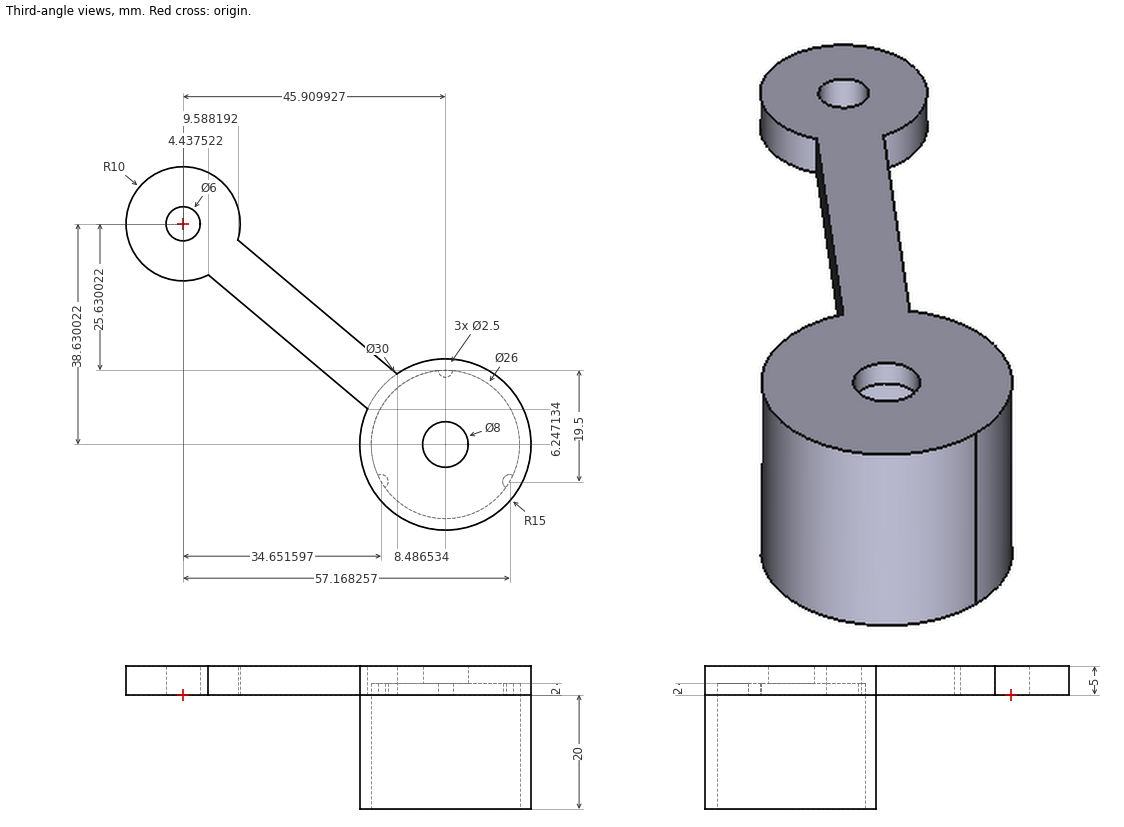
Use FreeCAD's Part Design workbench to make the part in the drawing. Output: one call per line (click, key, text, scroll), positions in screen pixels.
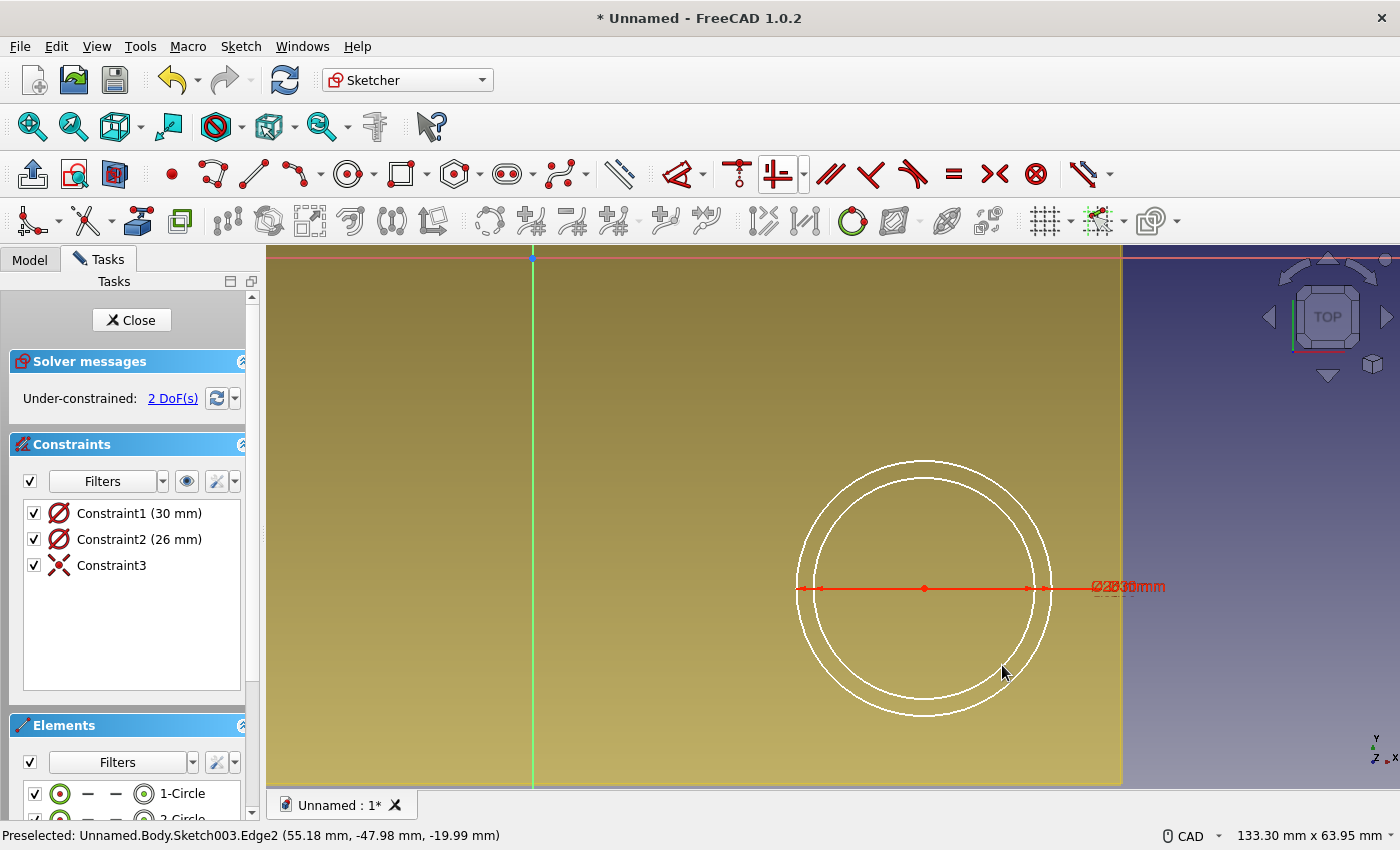
key(d)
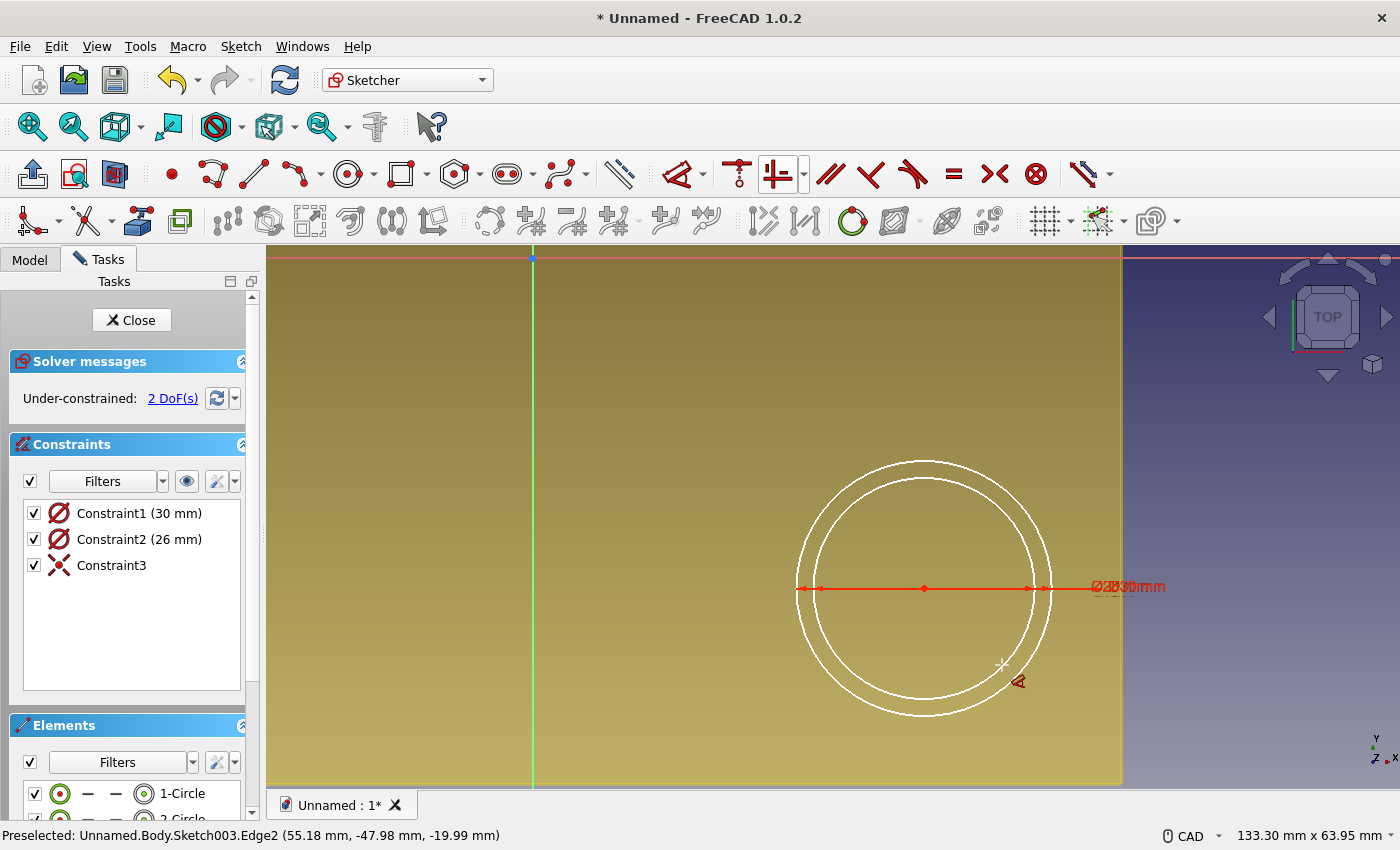
click(924, 589)
click(729, 623)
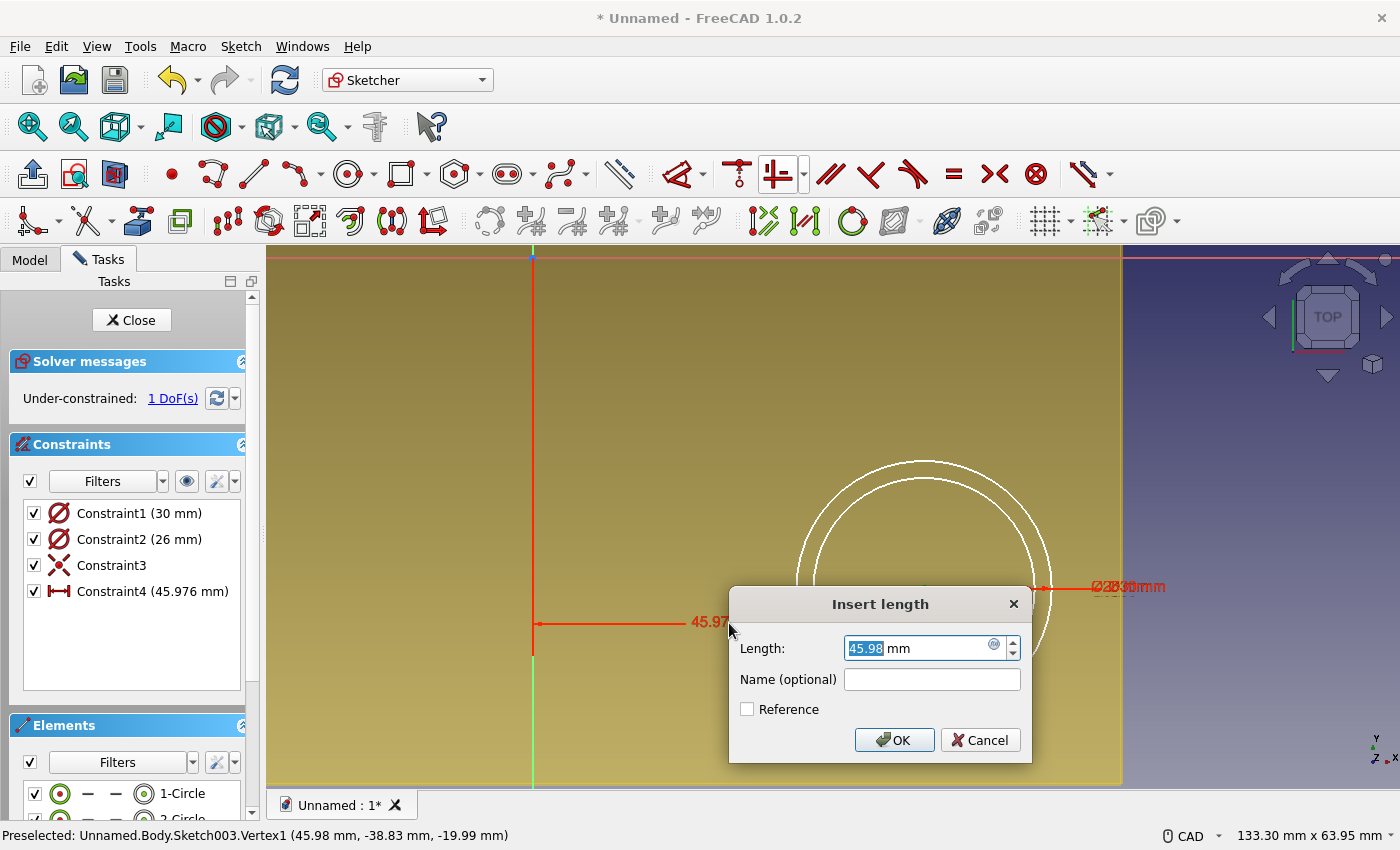
text(45.909927)
key(Return)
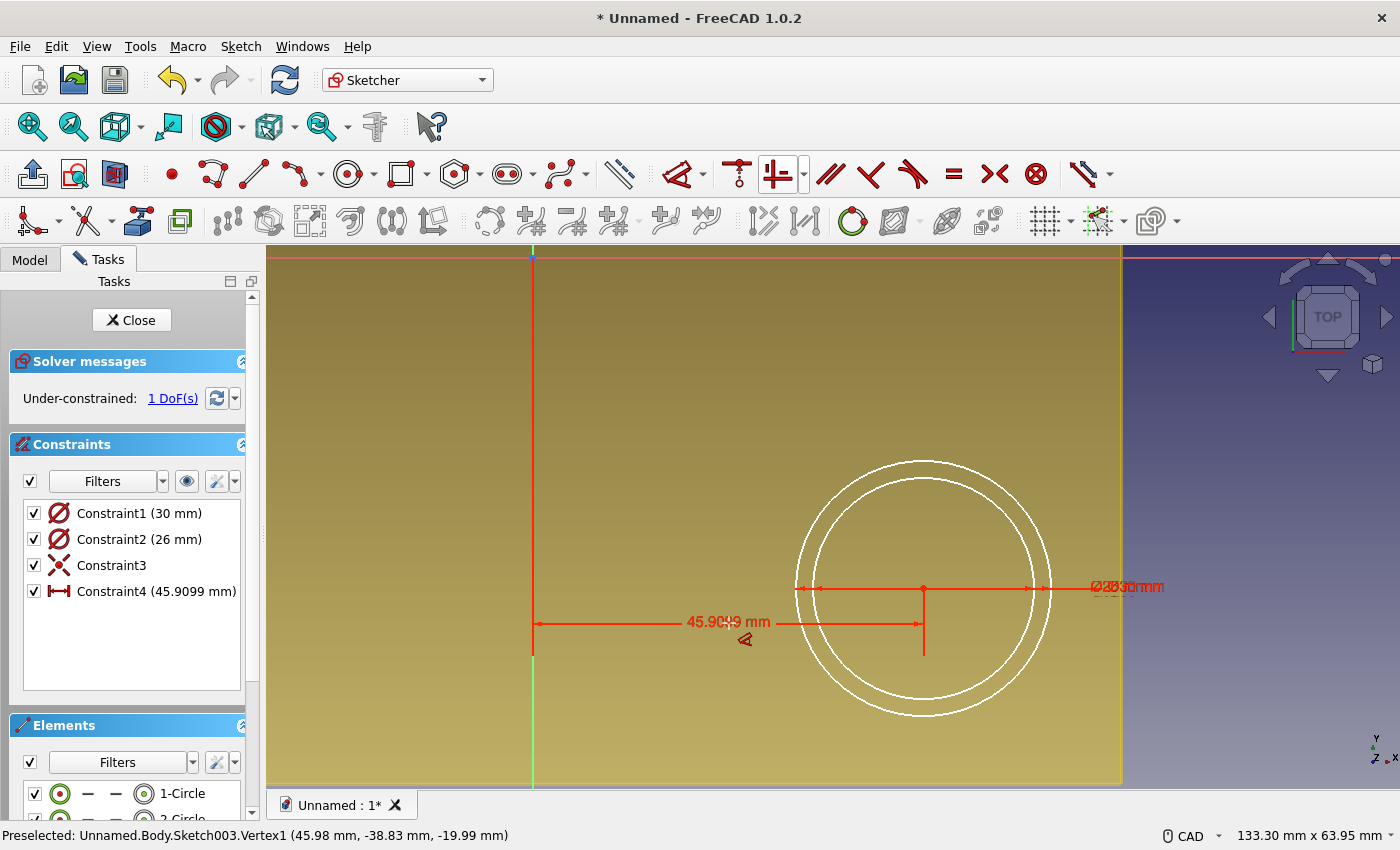
click(924, 589)
click(499, 431)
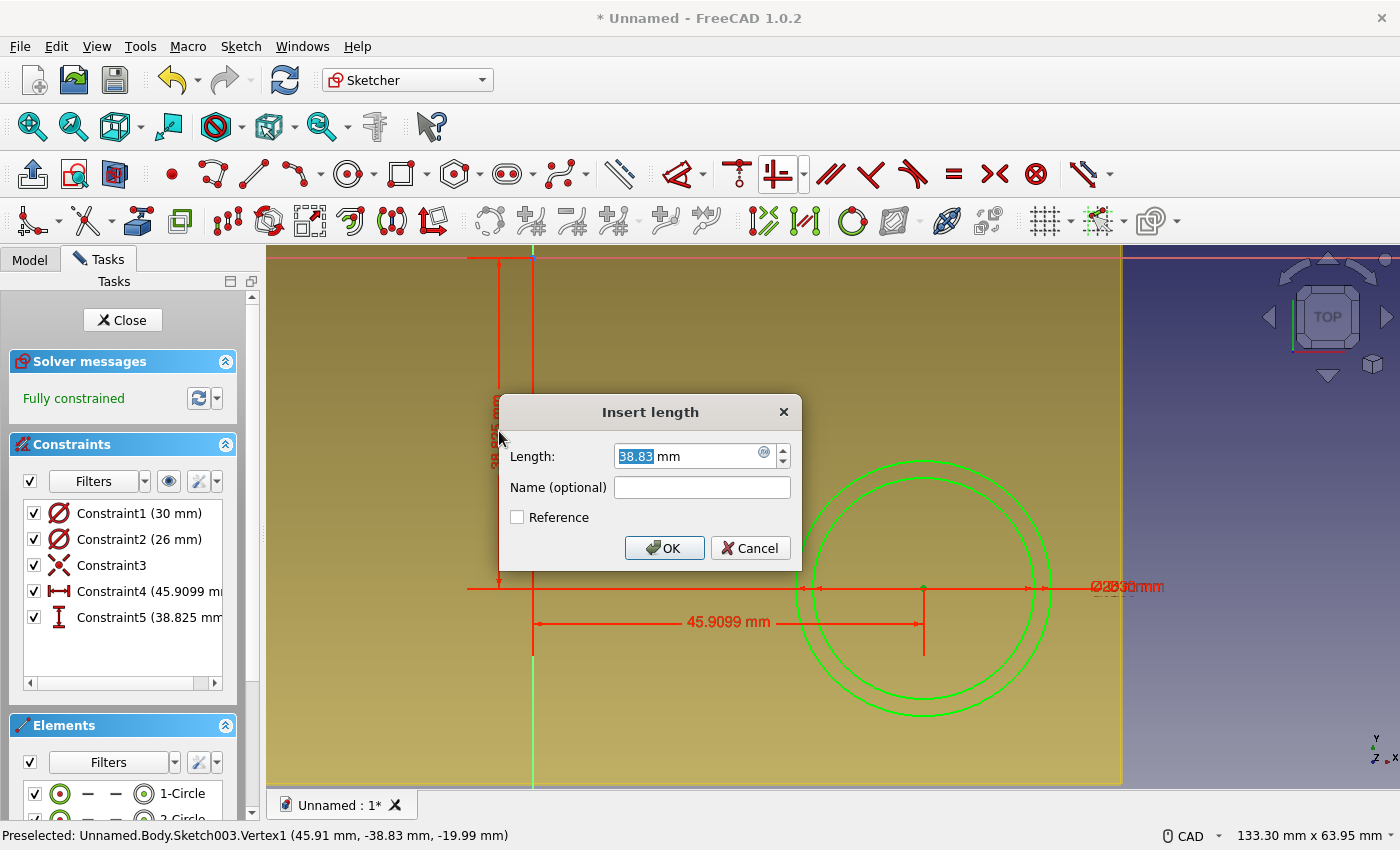
text(38.630022)
key(Return)
key(Escape)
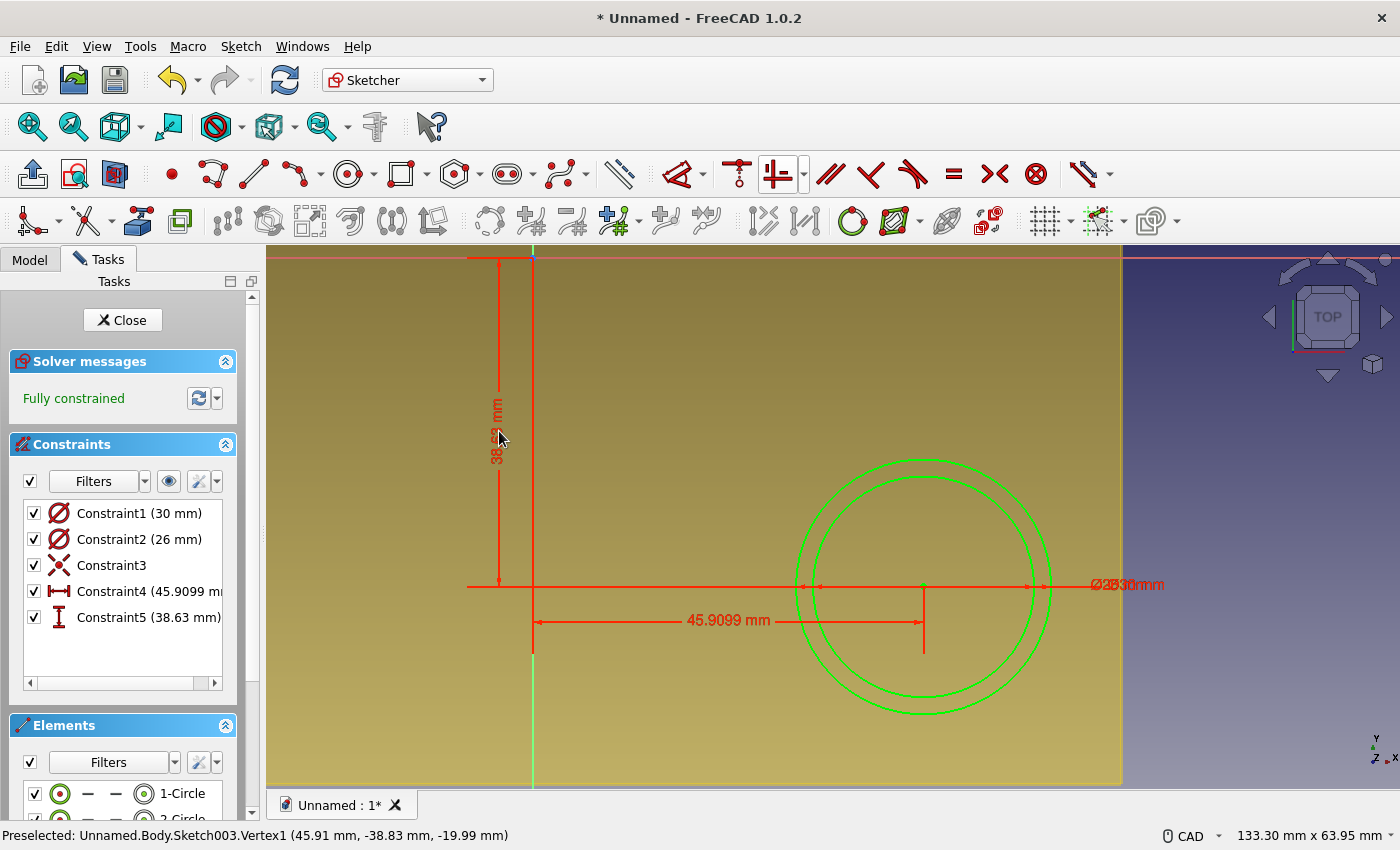
click(123, 320)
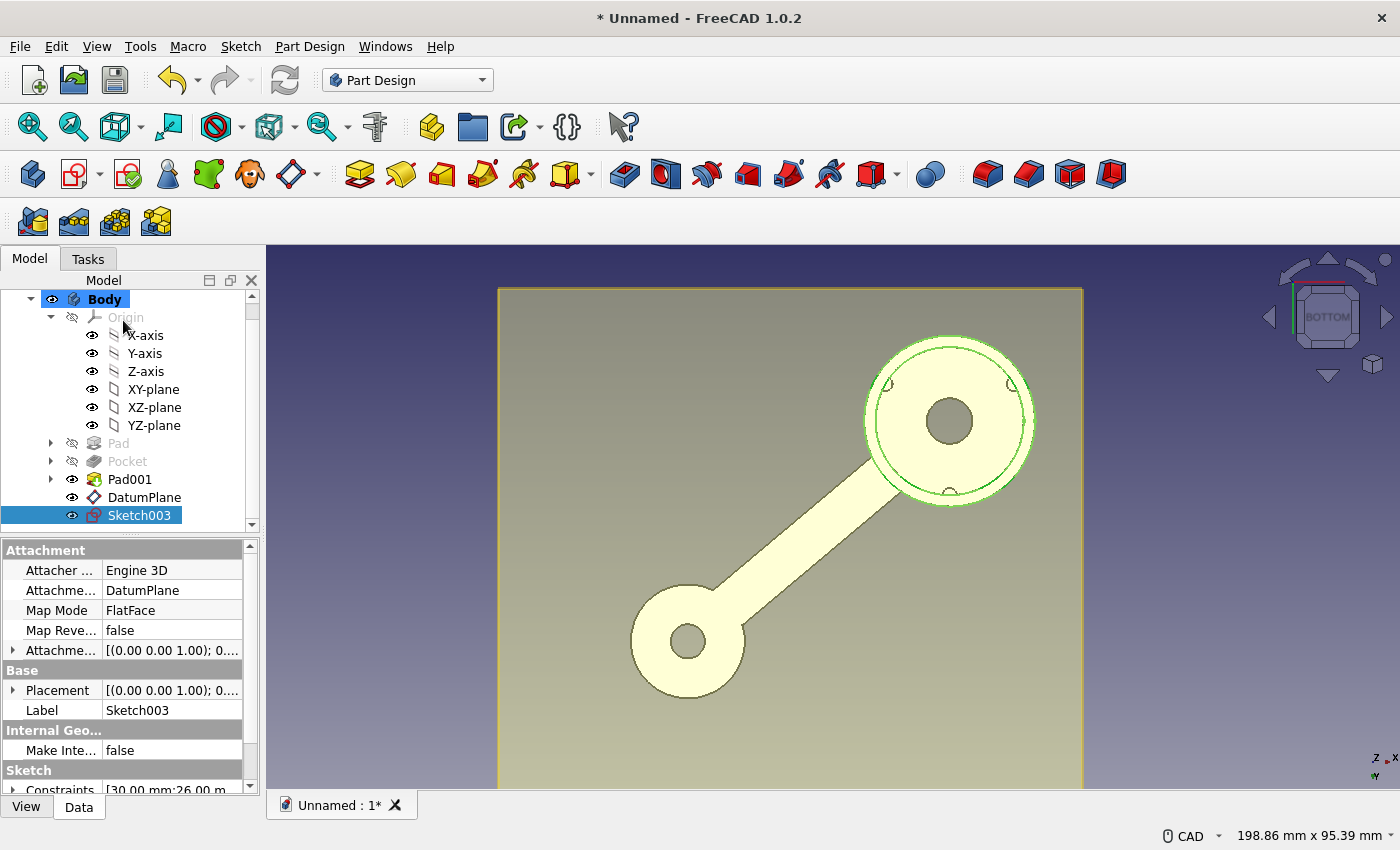
click(360, 174)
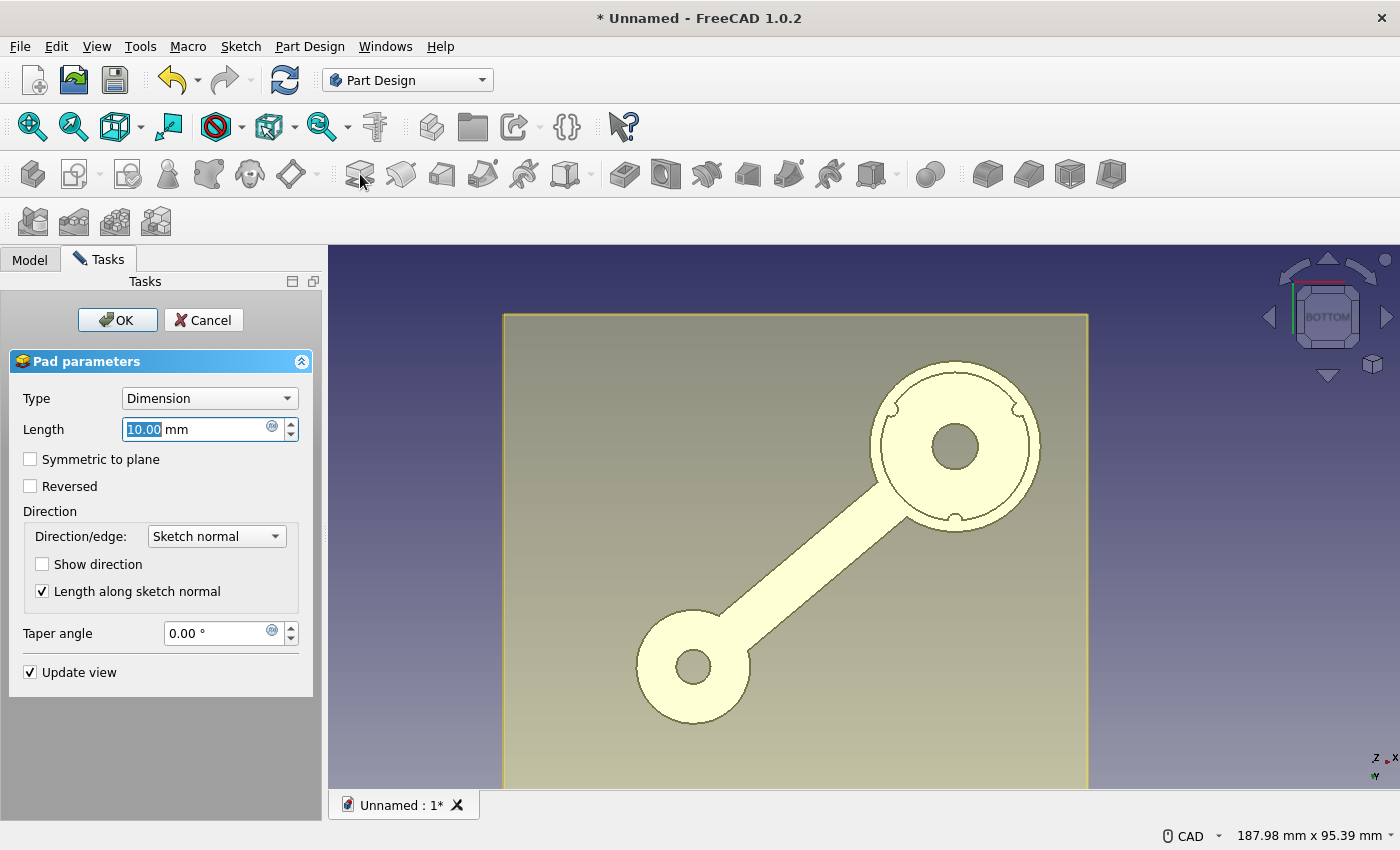
text(20)
key(Tab)